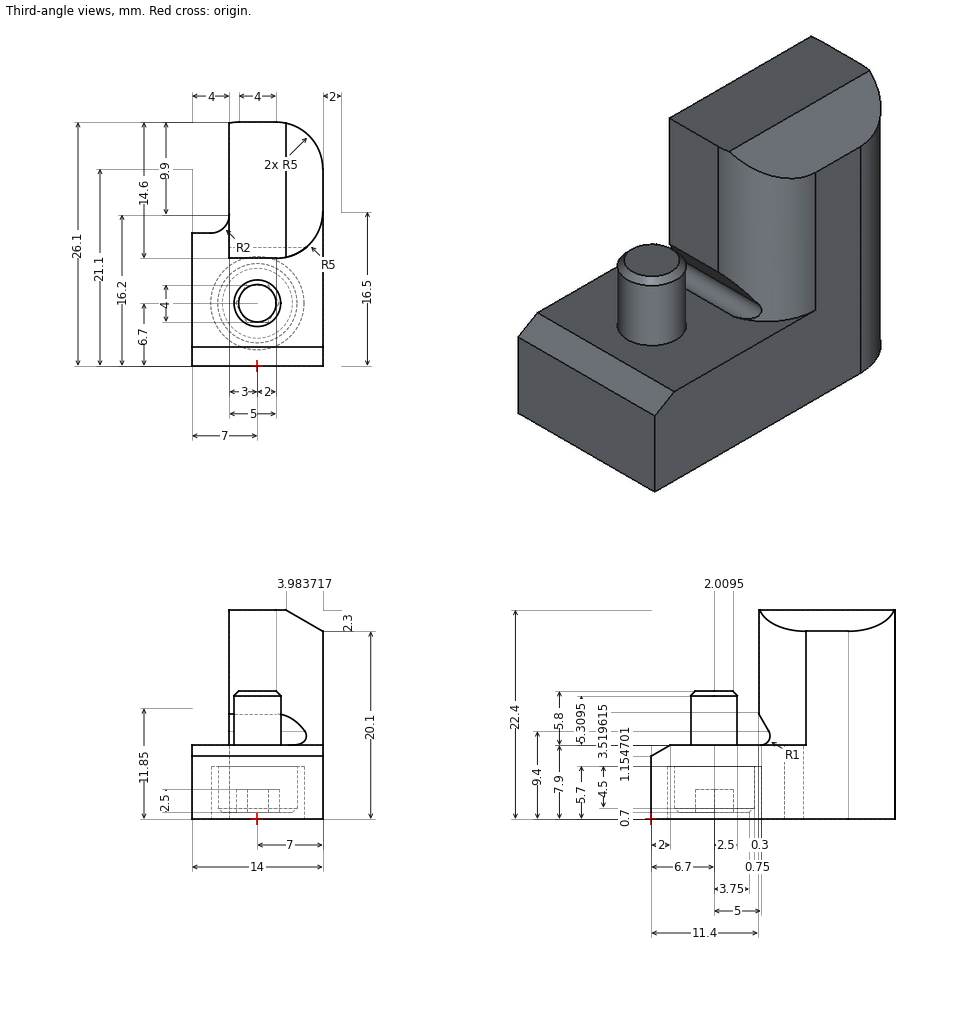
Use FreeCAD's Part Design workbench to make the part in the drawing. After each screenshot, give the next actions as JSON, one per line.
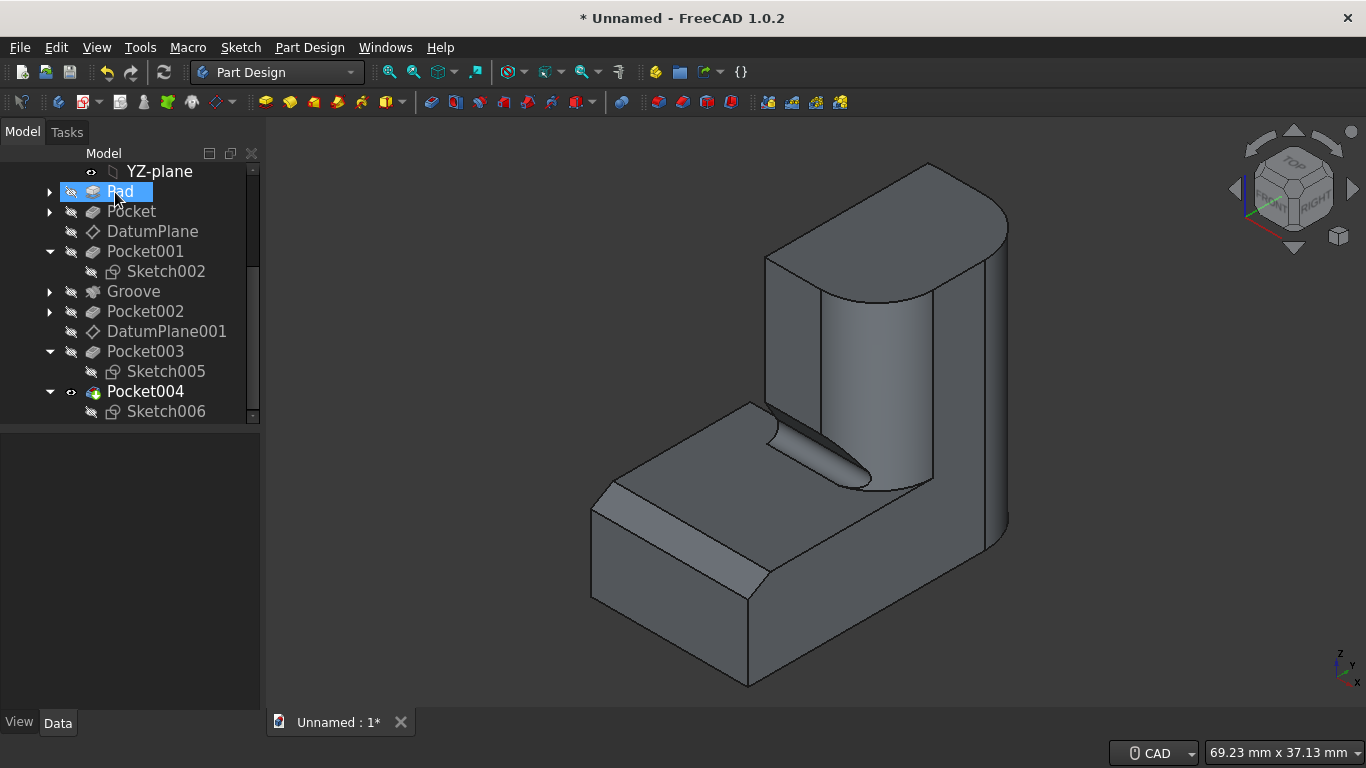
{"action": "left_click", "coordinate": [692, 610]}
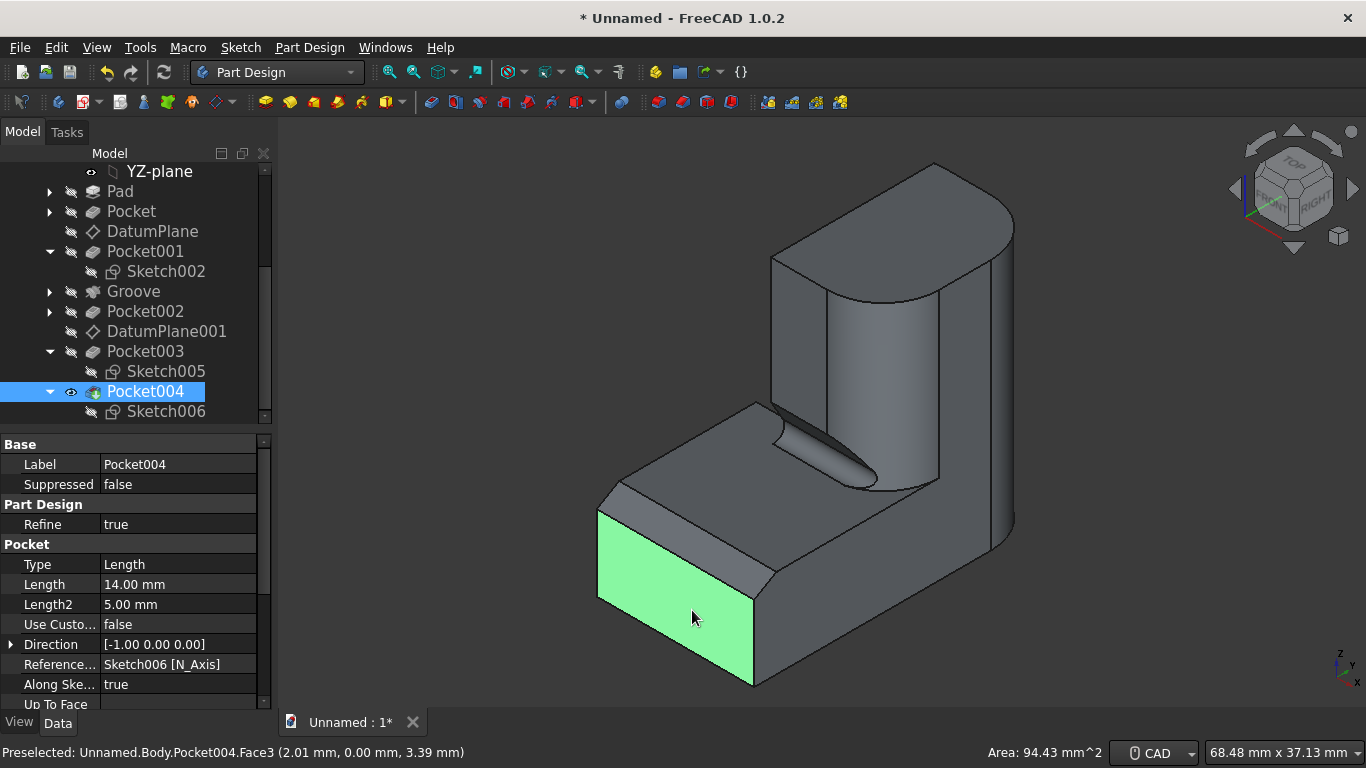
{"action": "left_click", "coordinate": [84, 102]}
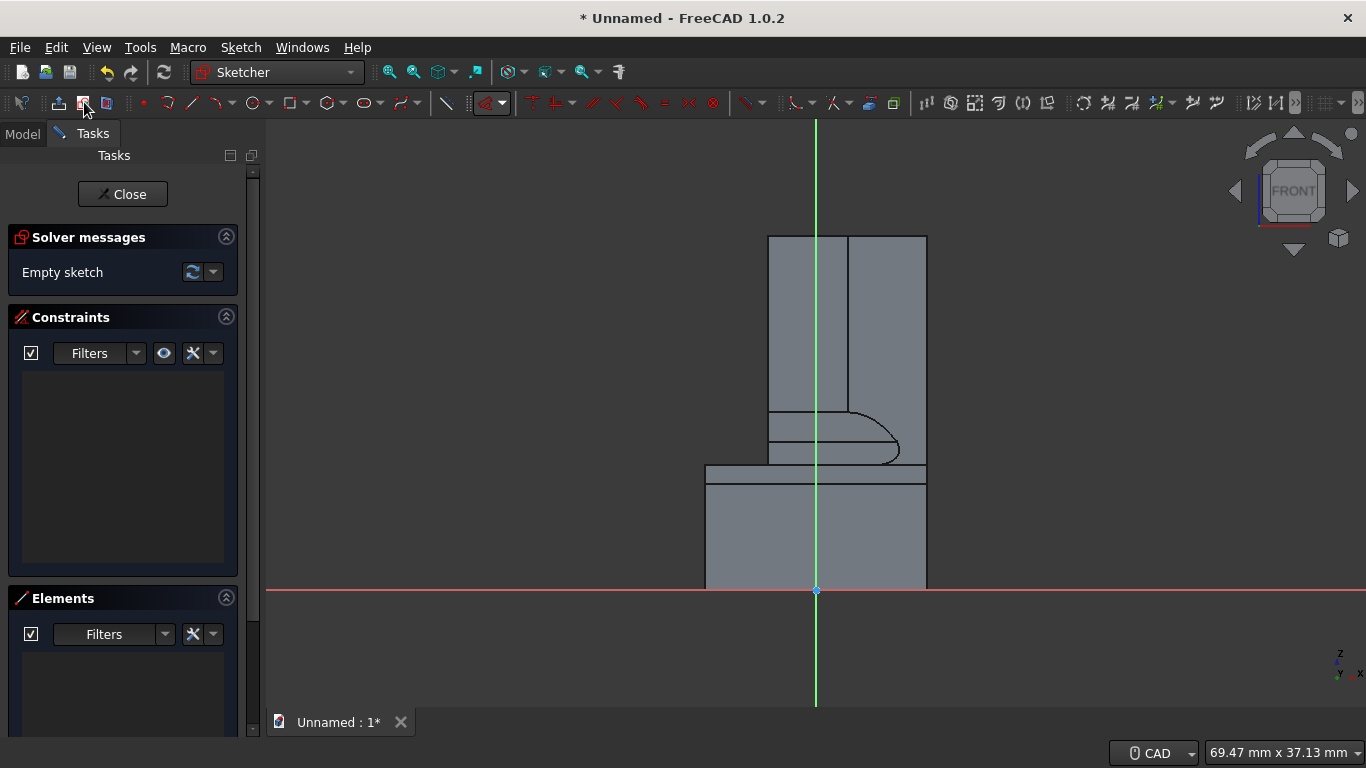
{"action": "scroll", "coordinate": [910, 238], "scroll_direction": "up", "scroll_amount": 12}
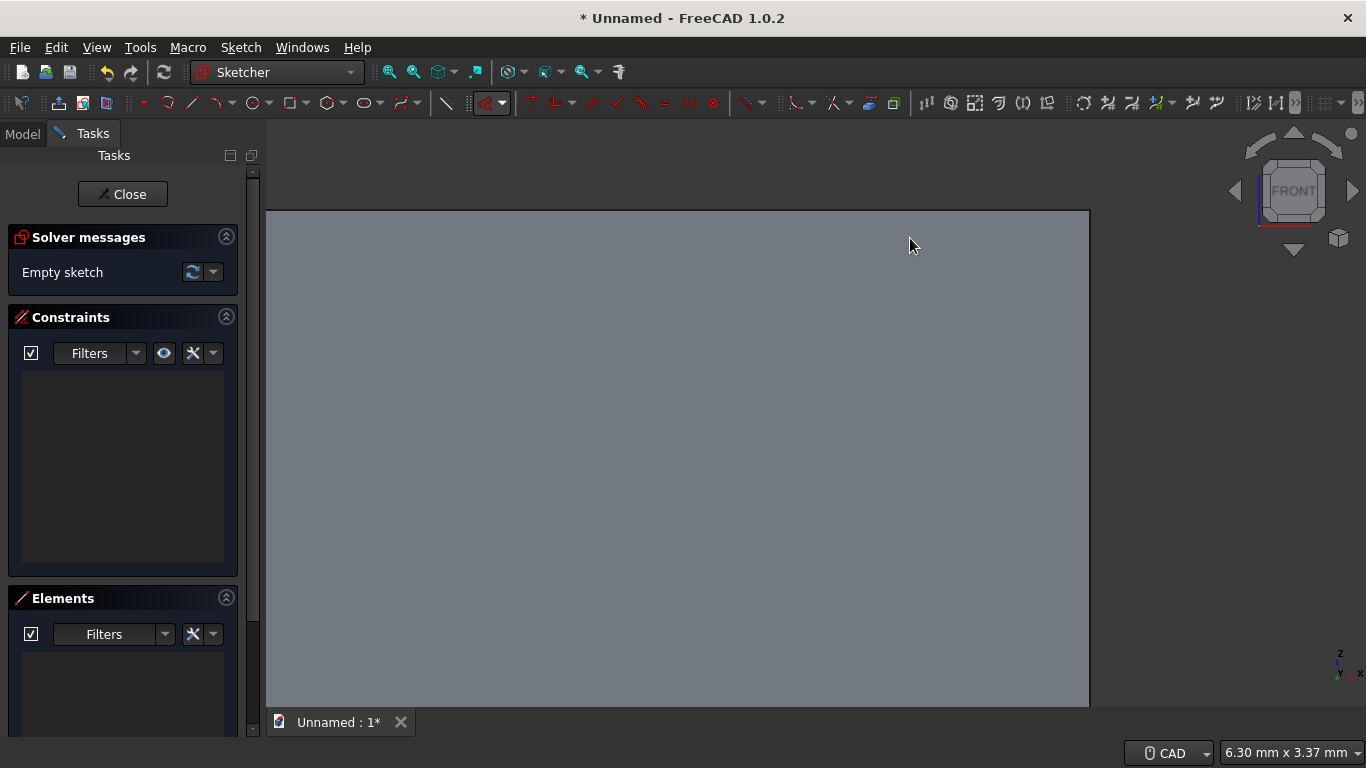
{"action": "left_click", "coordinate": [168, 104]}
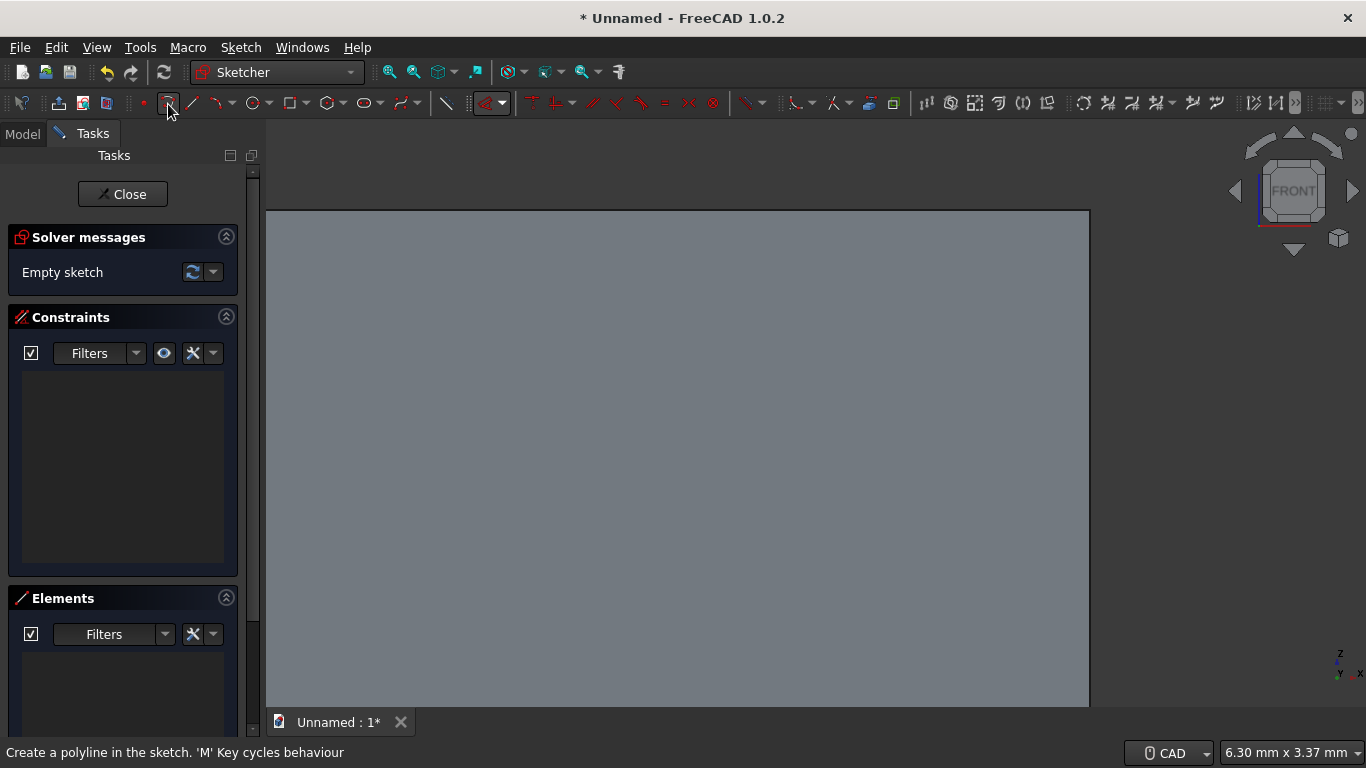
{"action": "left_click", "coordinate": [1090, 612]}
{"action": "left_click", "coordinate": [394, 210]}
{"action": "left_click", "coordinate": [1090, 210]}
{"action": "left_click", "coordinate": [1090, 613]}
{"action": "key", "text": "Escape"}
{"action": "key", "text": "Escape"}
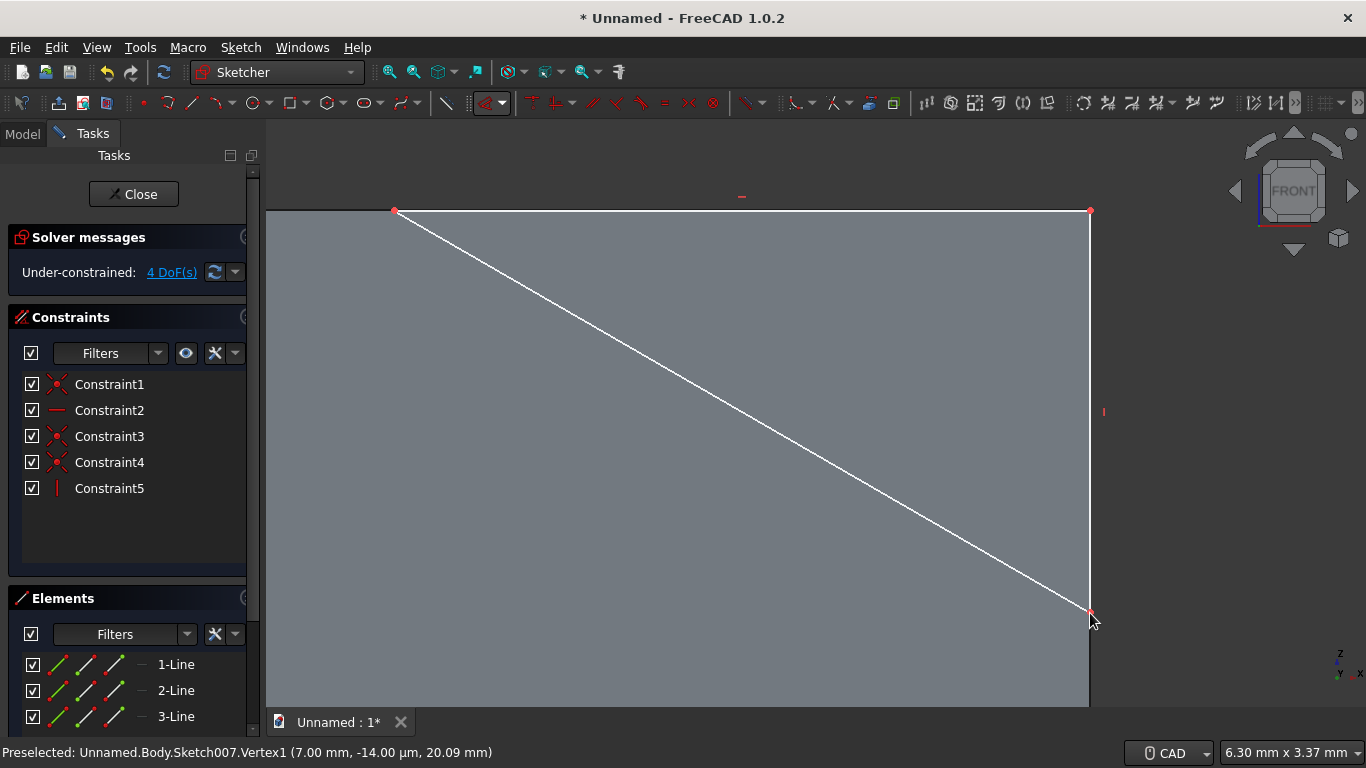
{"action": "left_click", "coordinate": [1090, 613]}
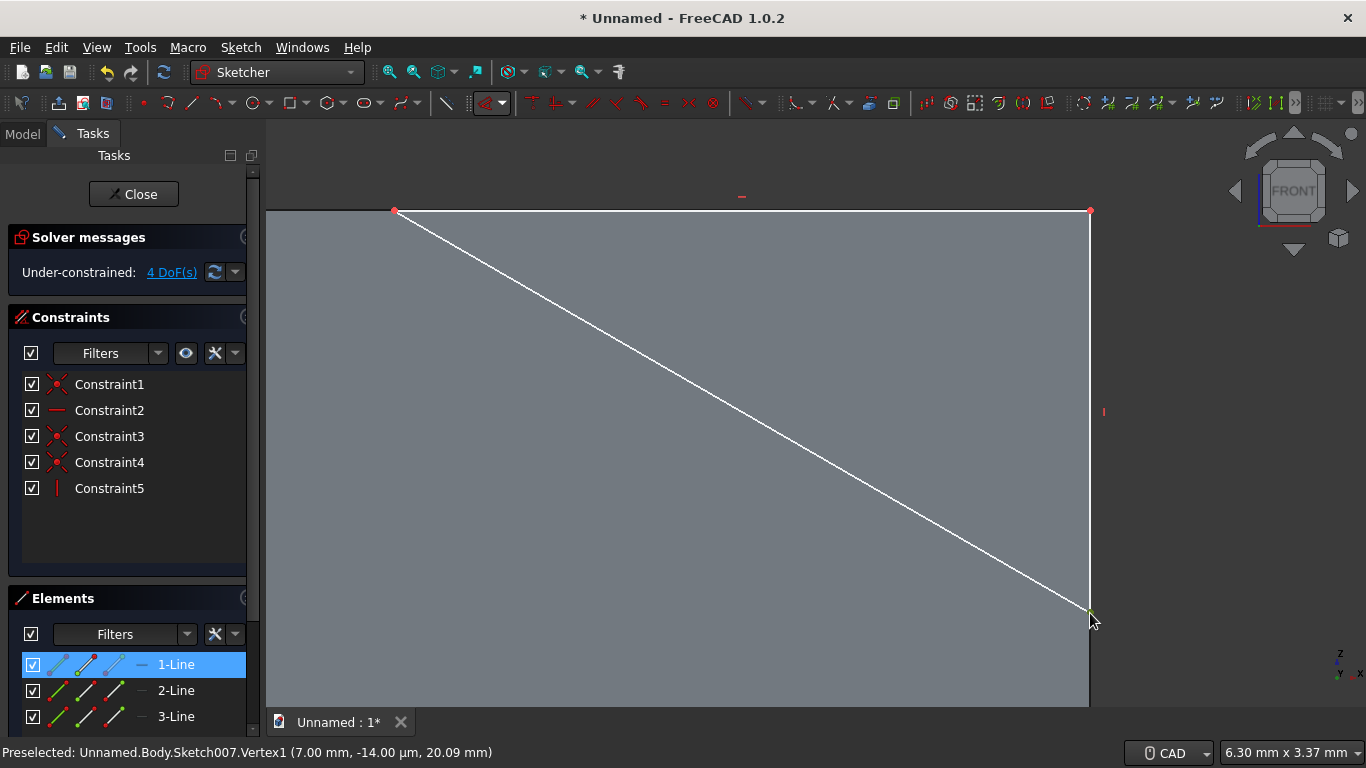
{"action": "key", "text": "l"}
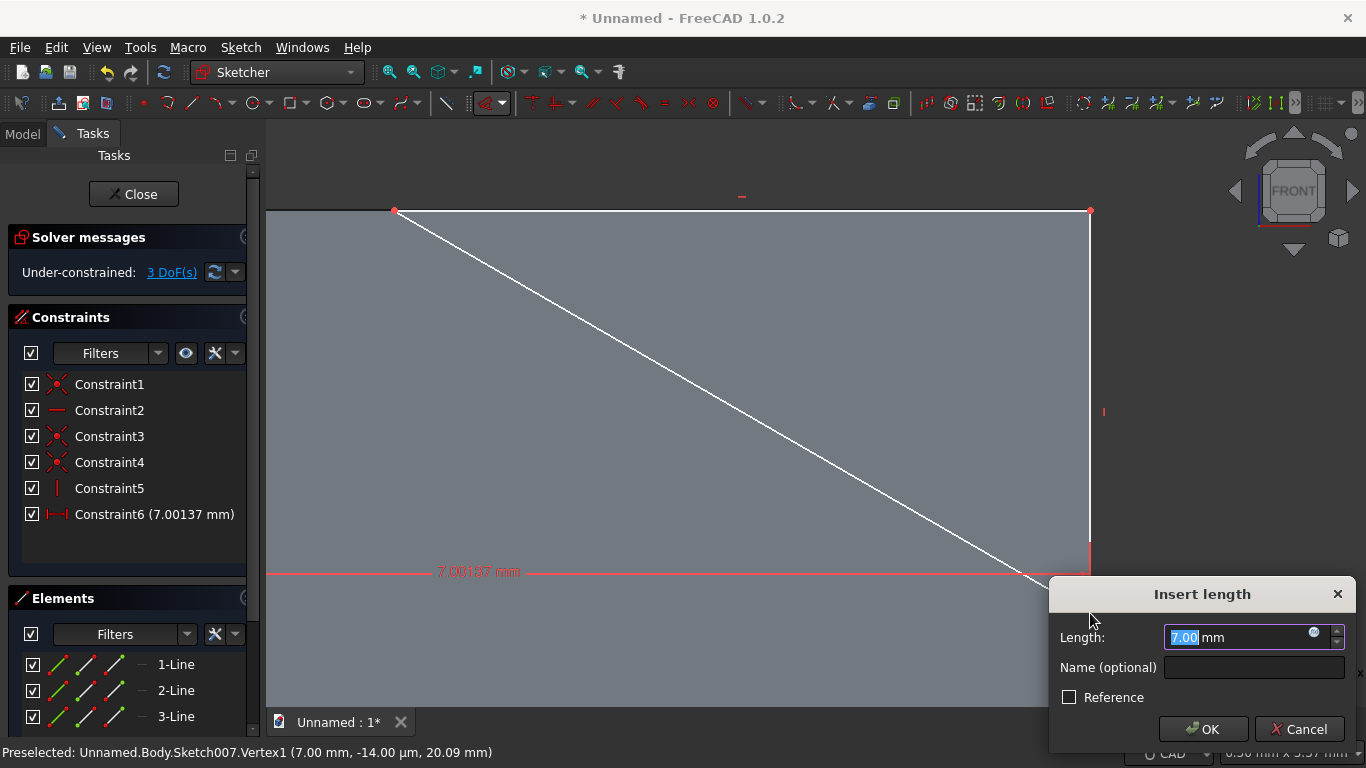
{"action": "type", "text": "7"}
{"action": "key", "text": "Return"}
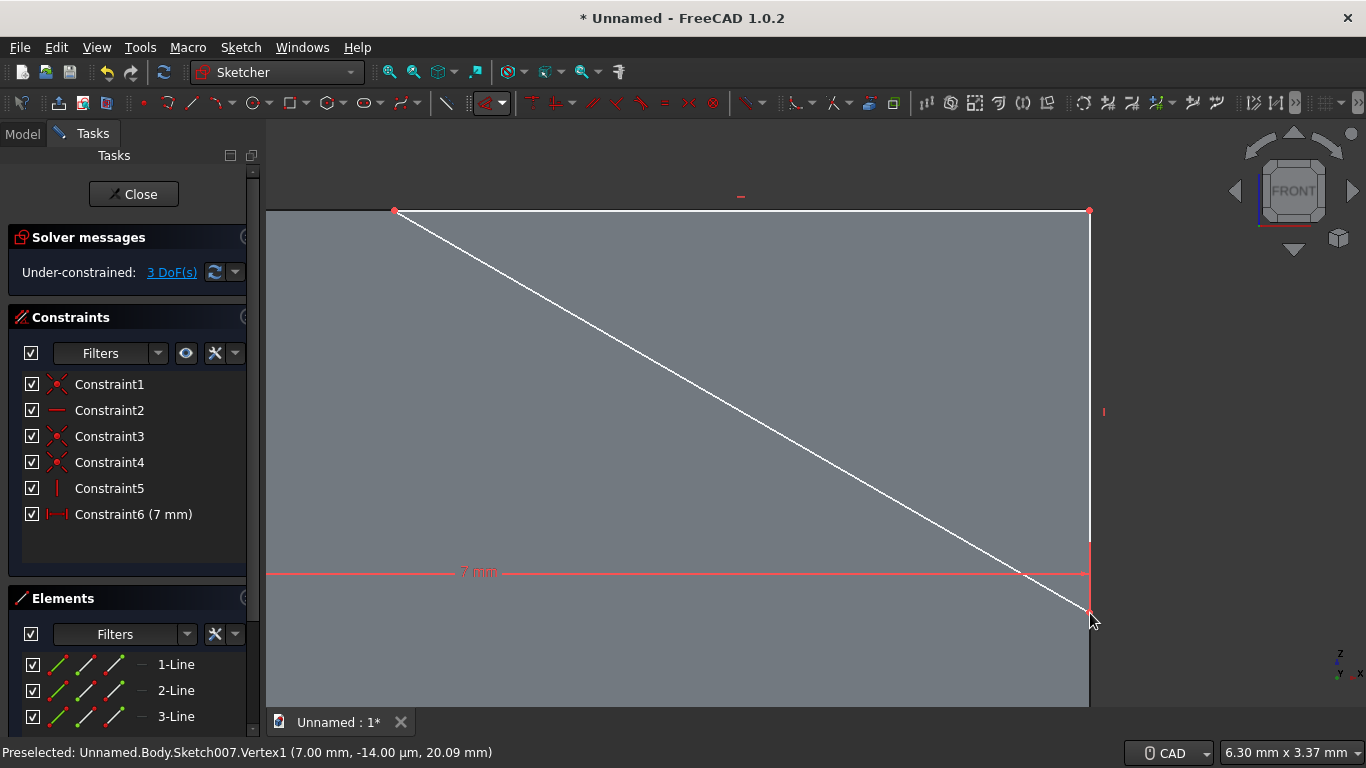
{"action": "left_click", "coordinate": [1090, 332]}